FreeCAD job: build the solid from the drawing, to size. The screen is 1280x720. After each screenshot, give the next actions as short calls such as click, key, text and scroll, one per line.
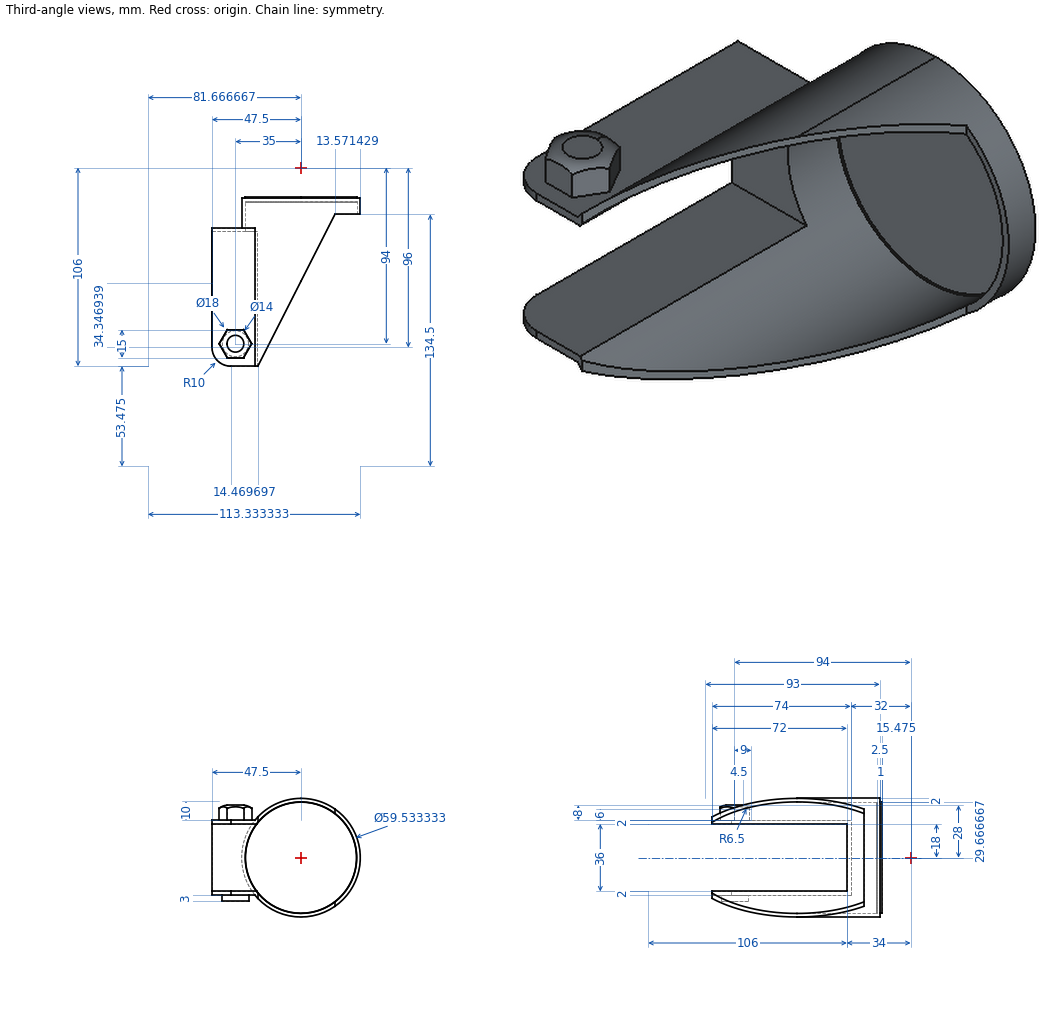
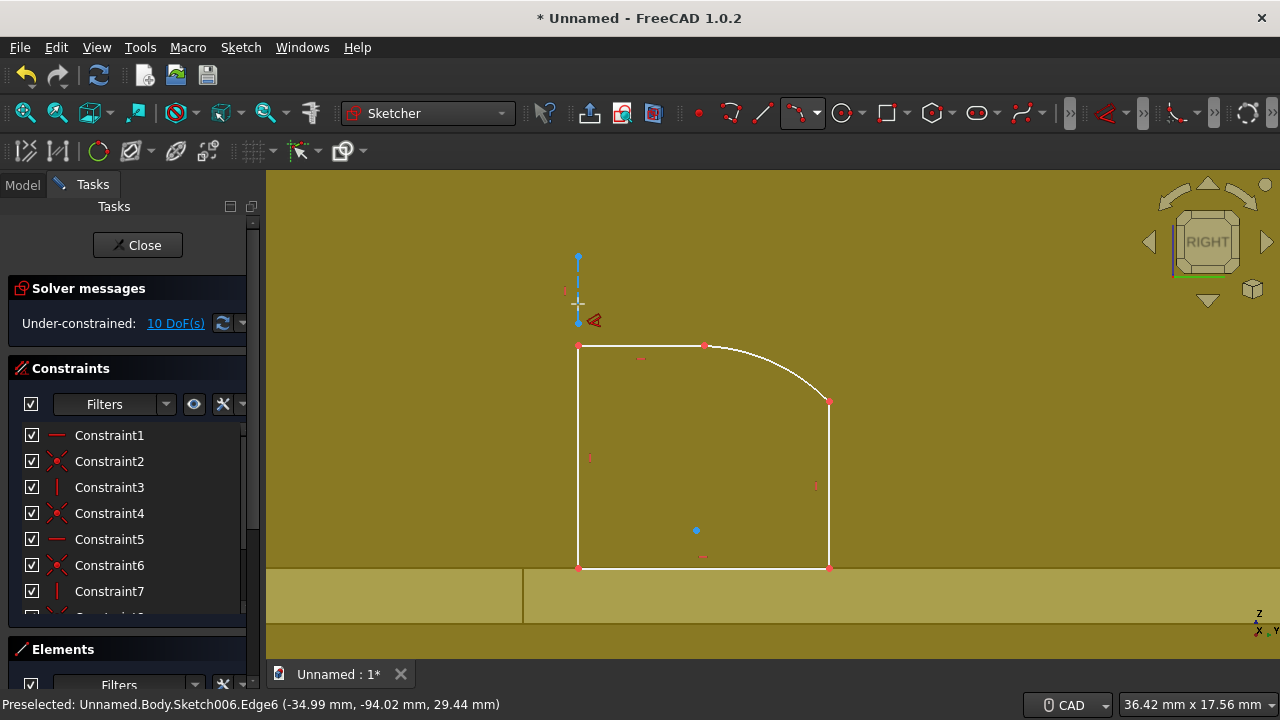
click(797, 375)
click(814, 348)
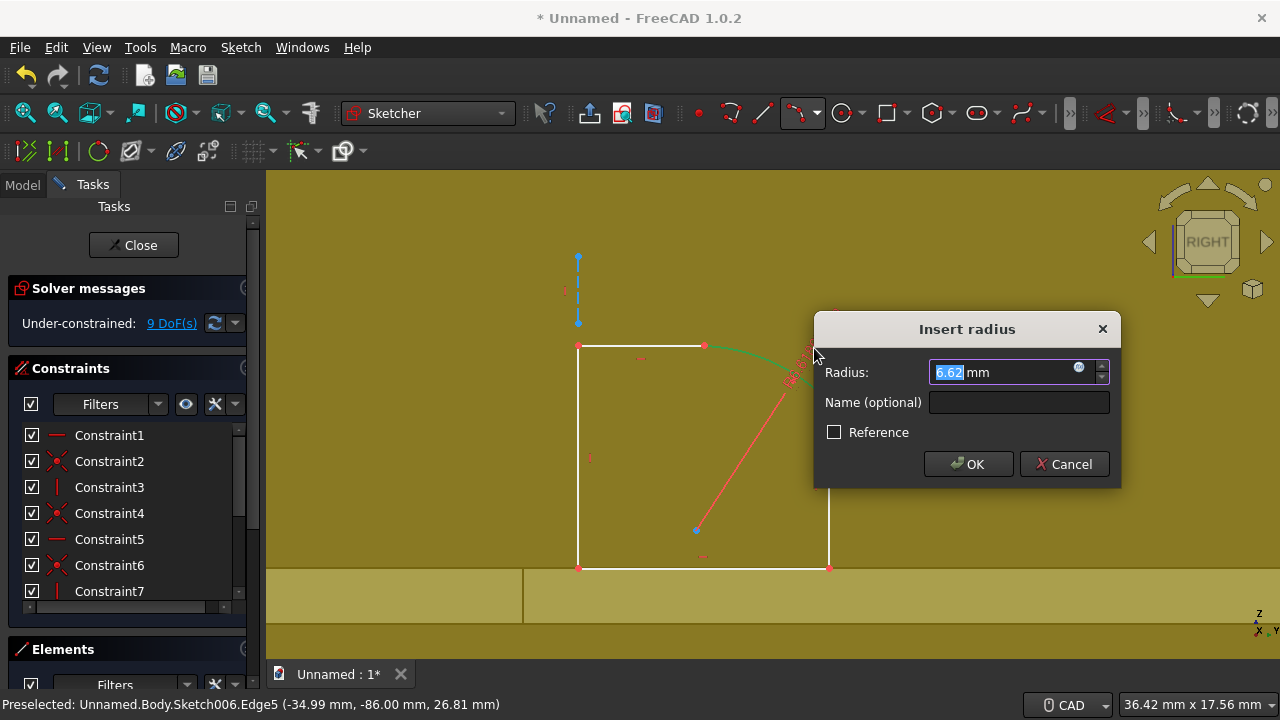
text(6.5)
key(Return)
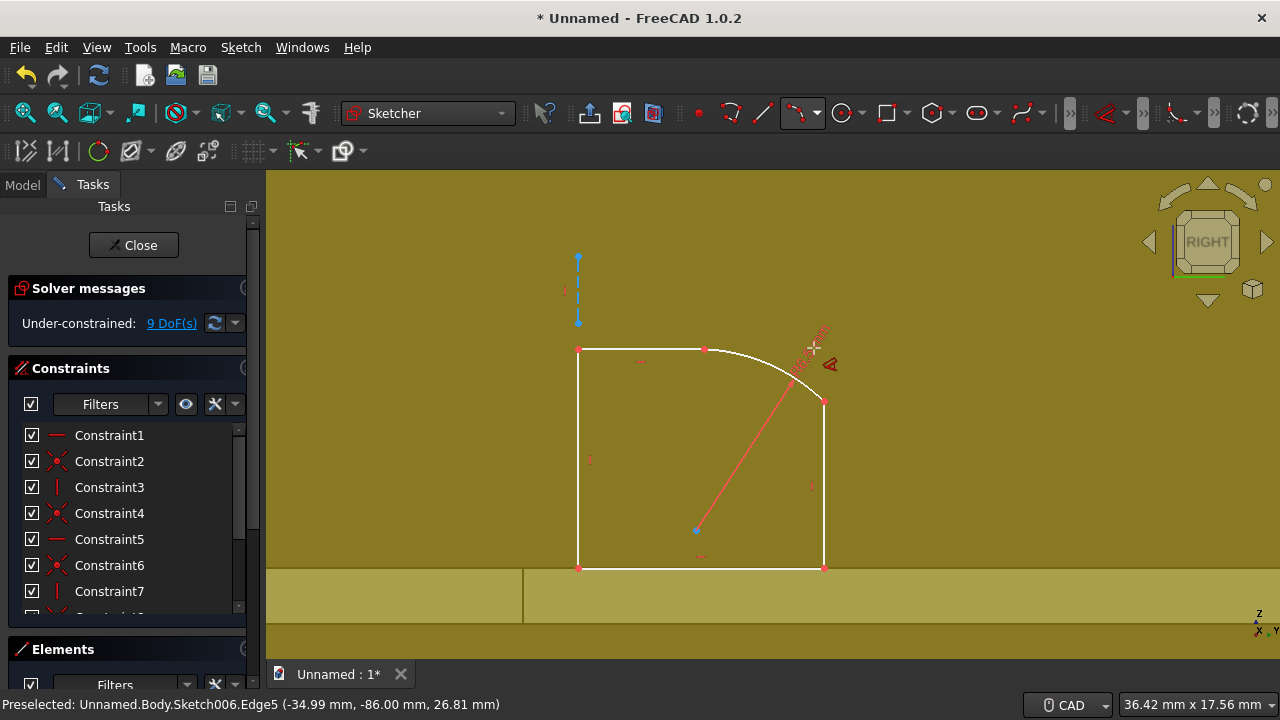
click(578, 415)
click(544, 459)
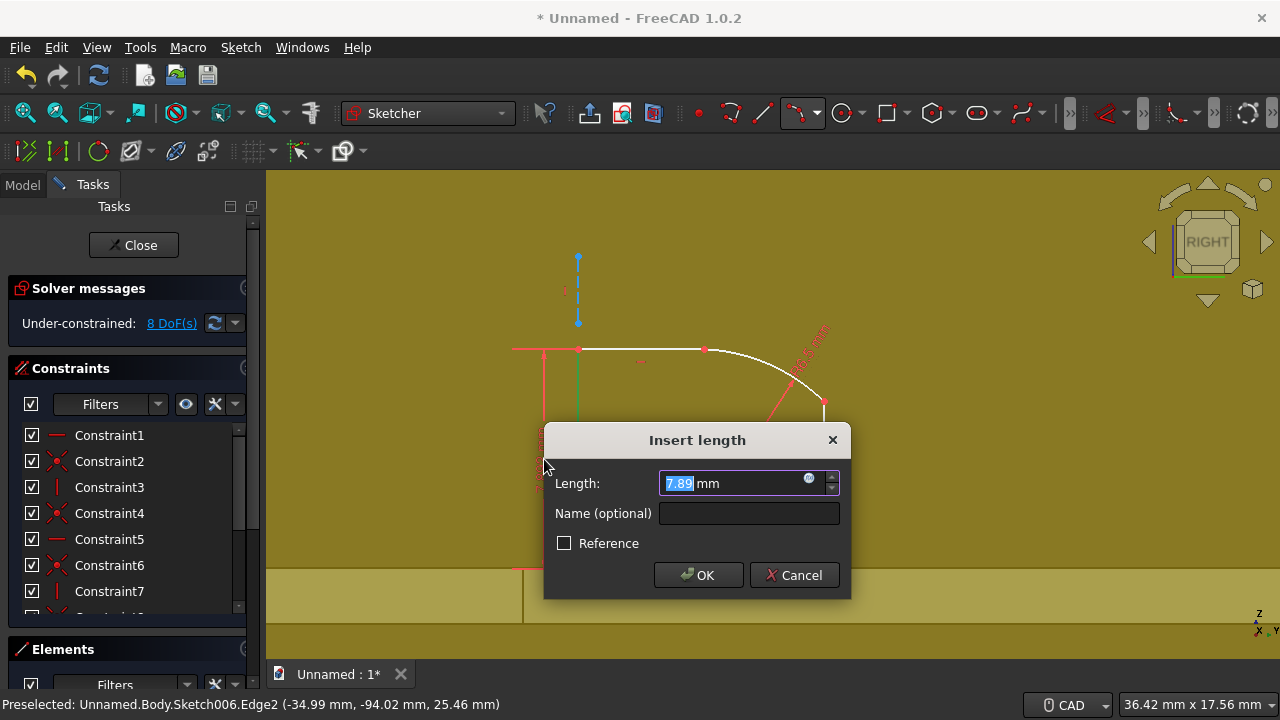
text(8)
key(Return)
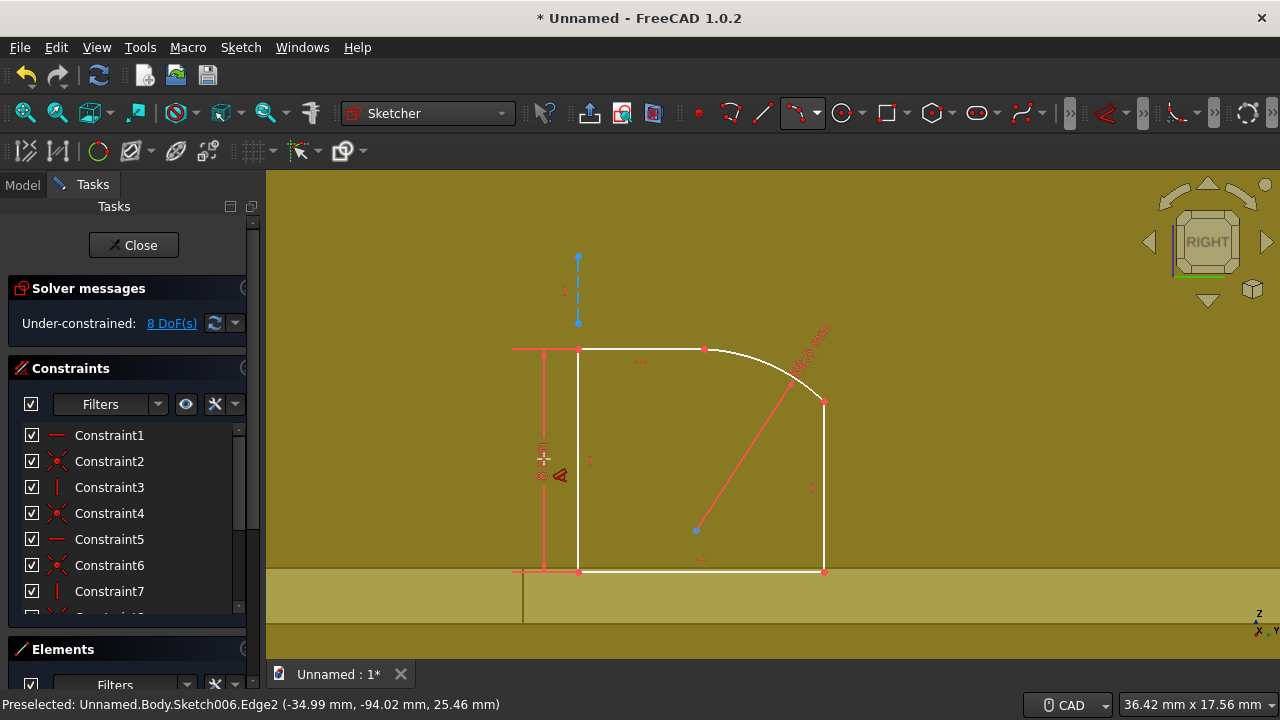
click(652, 572)
click(701, 606)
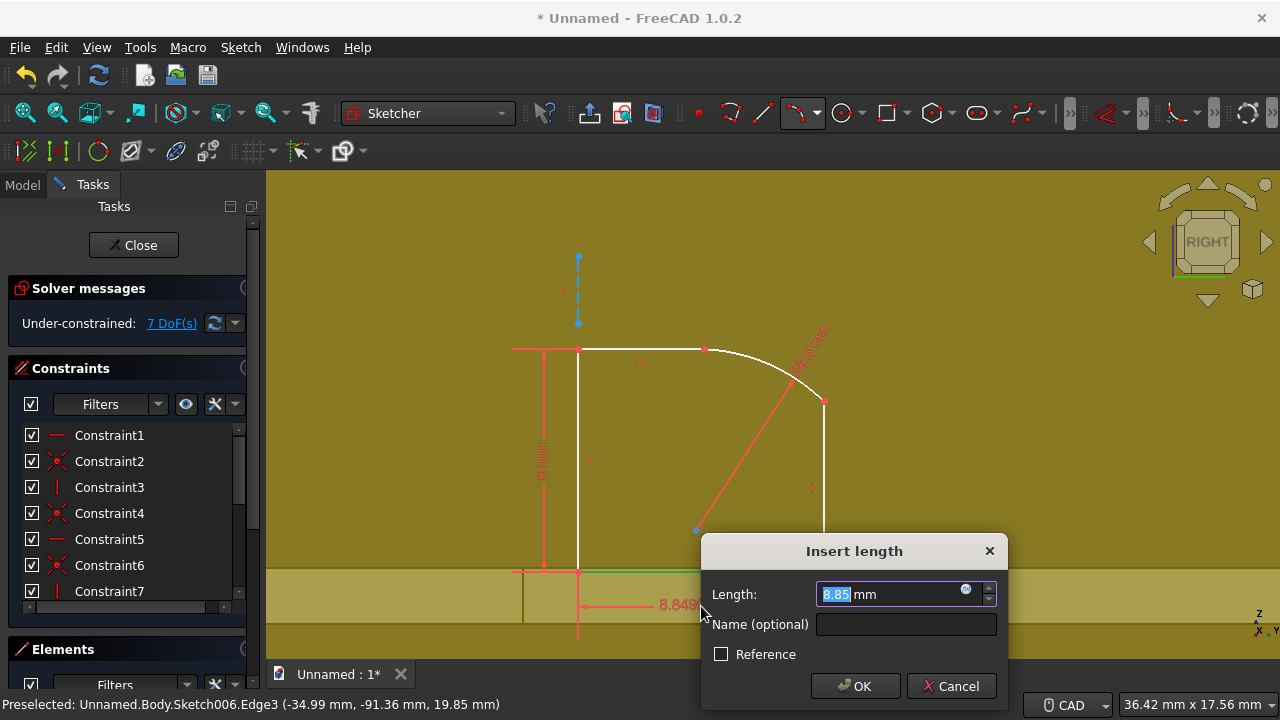
text(9)
key(Return)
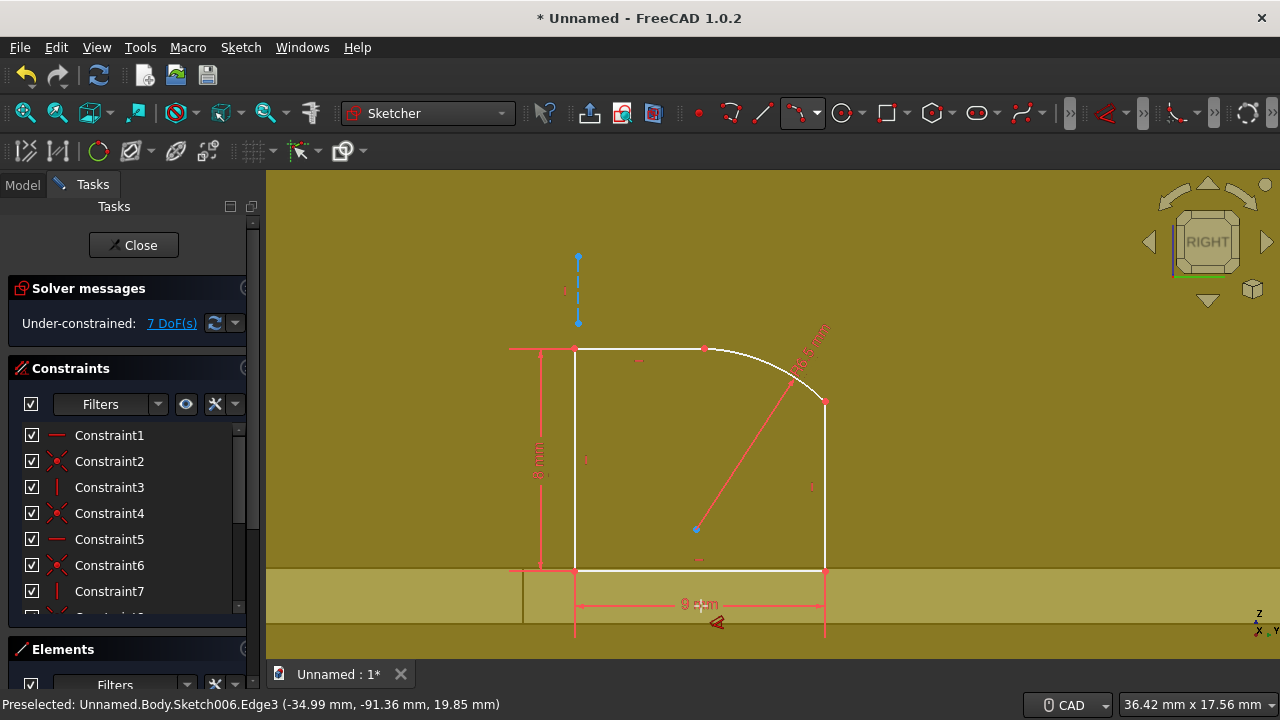
click(825, 521)
click(859, 487)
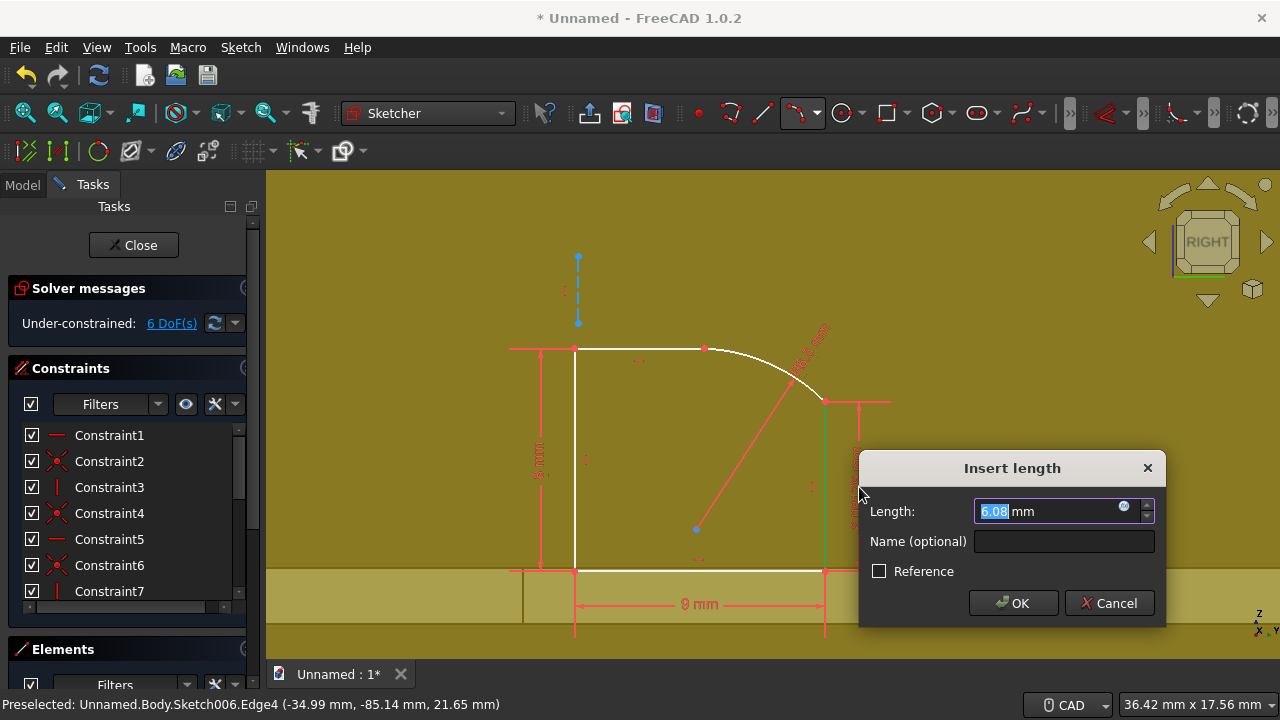
text(6)
key(Return)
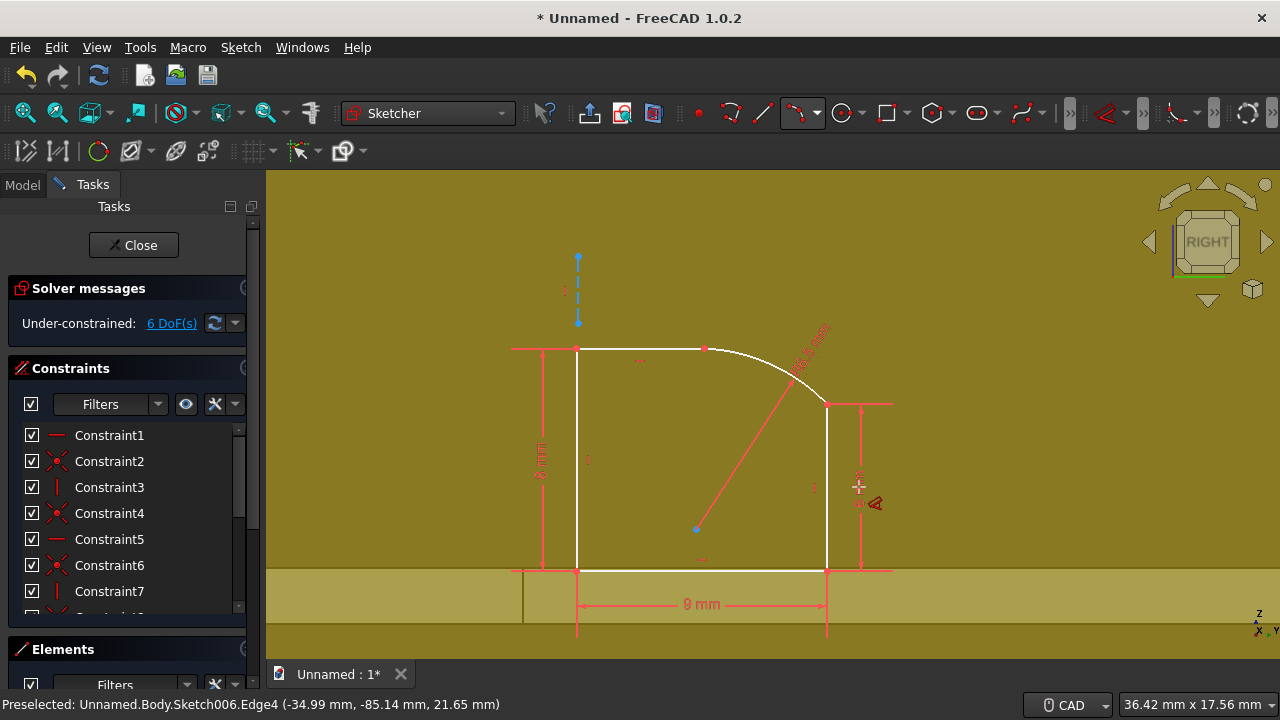
click(666, 349)
click(640, 315)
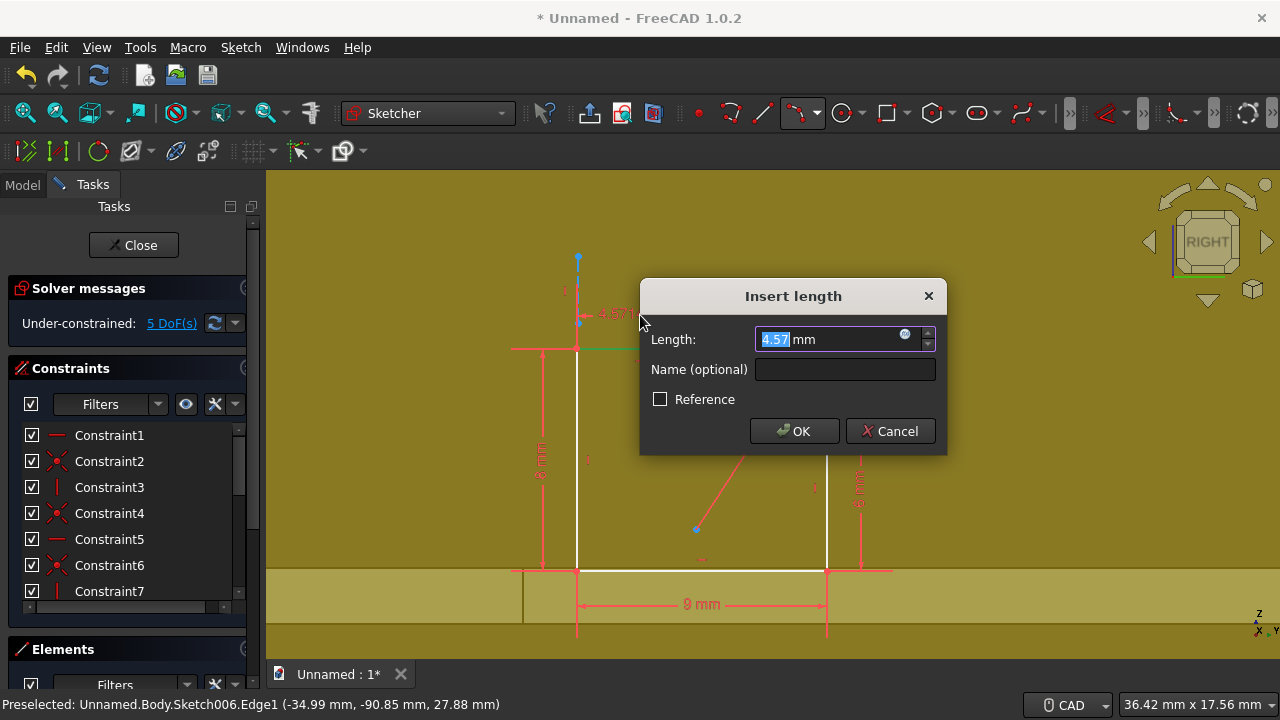
text(4.5)
key(Return)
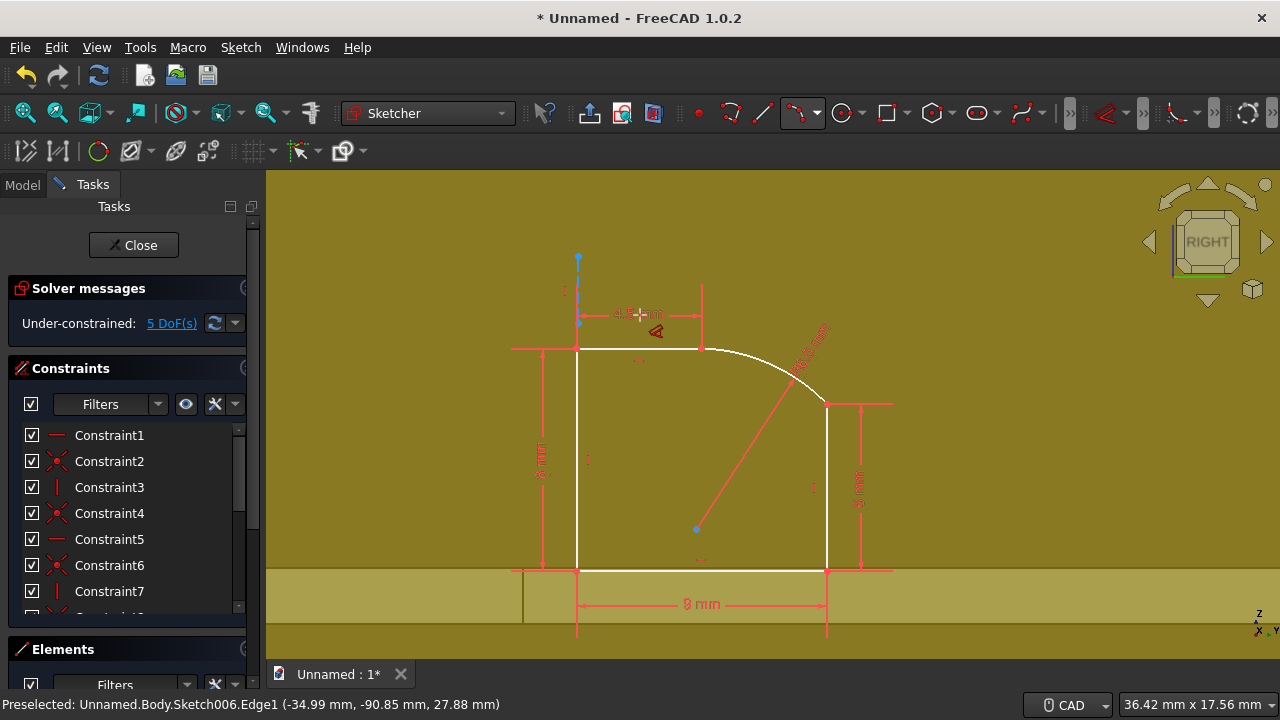
click(702, 349)
click(668, 490)